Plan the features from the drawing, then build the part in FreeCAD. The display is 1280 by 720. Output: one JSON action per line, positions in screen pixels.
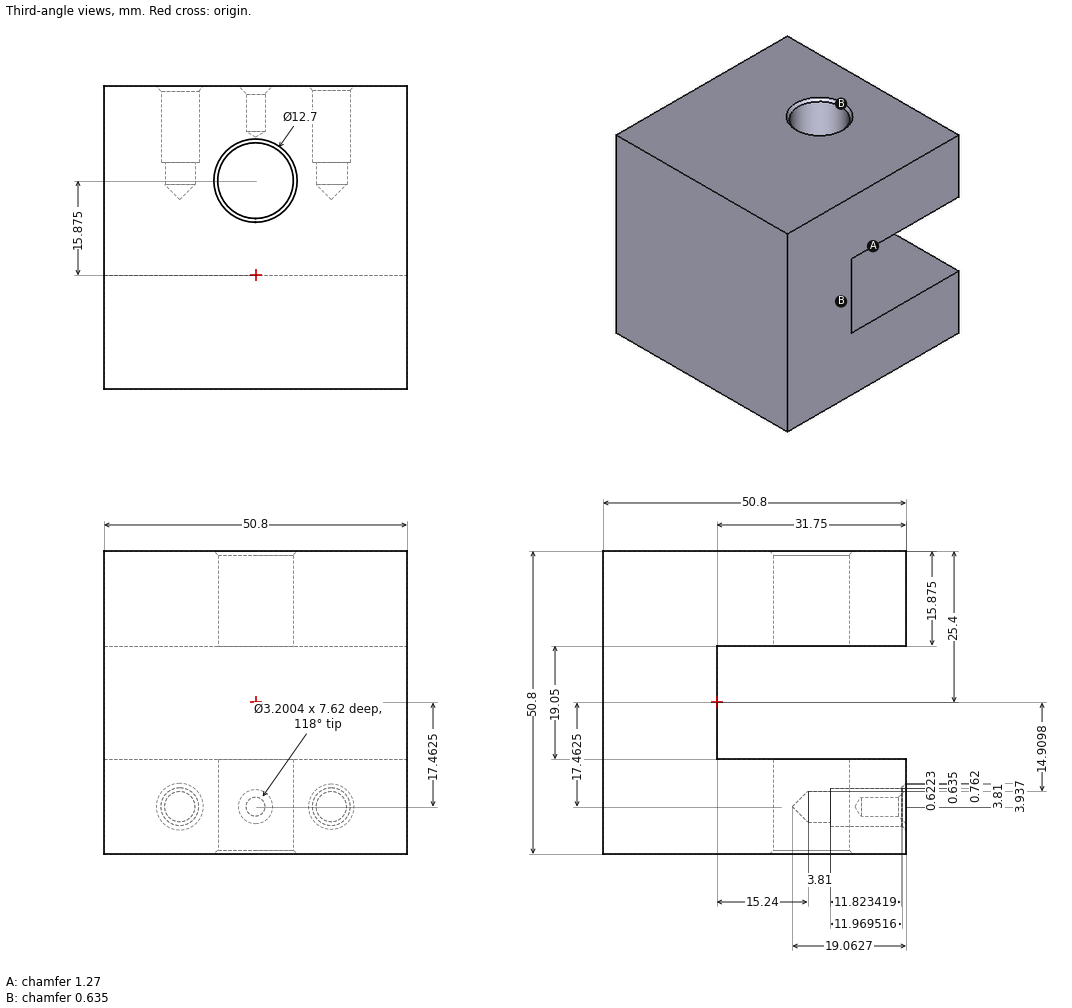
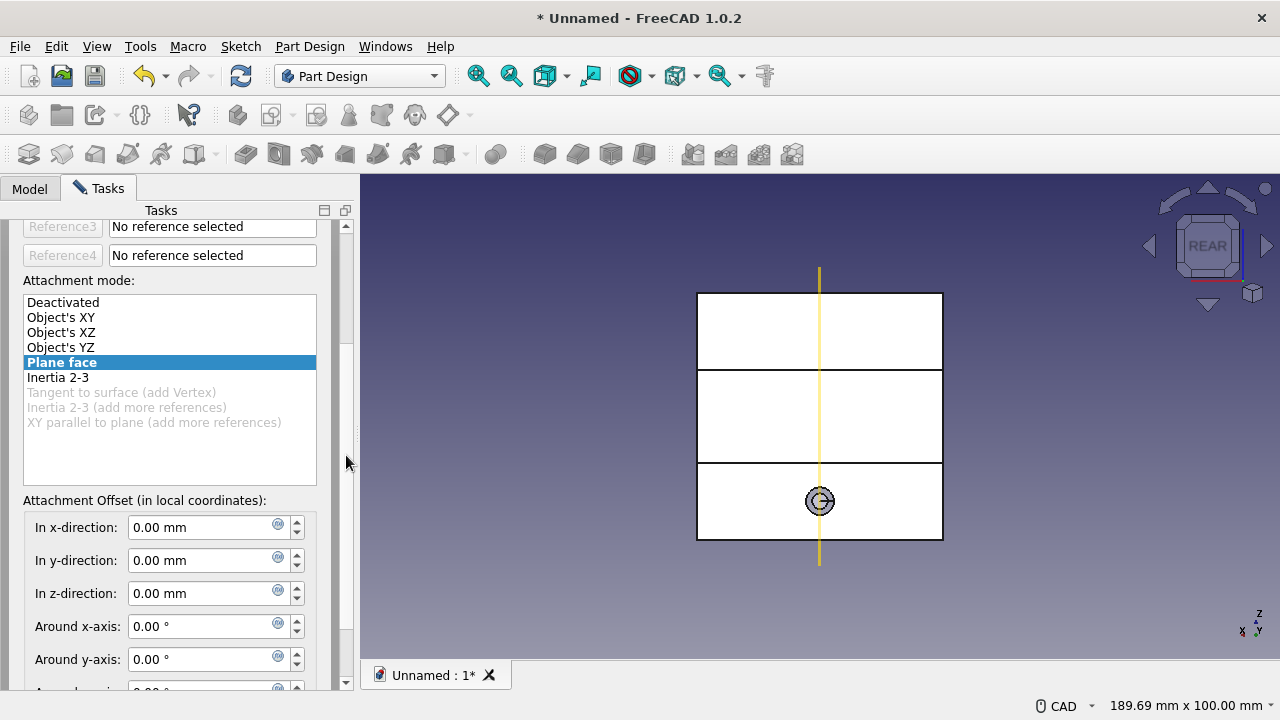
{"action": "triple_click", "coordinate": [210, 594]}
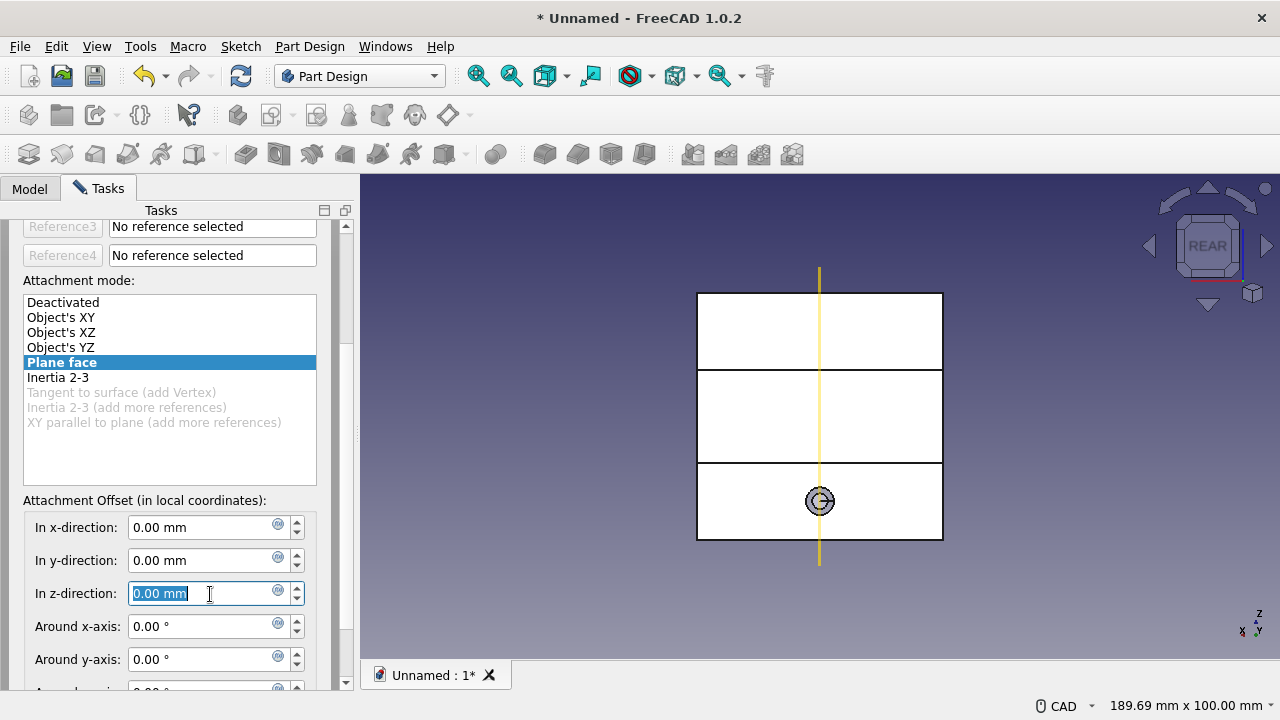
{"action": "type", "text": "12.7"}
{"action": "key", "text": "Tab"}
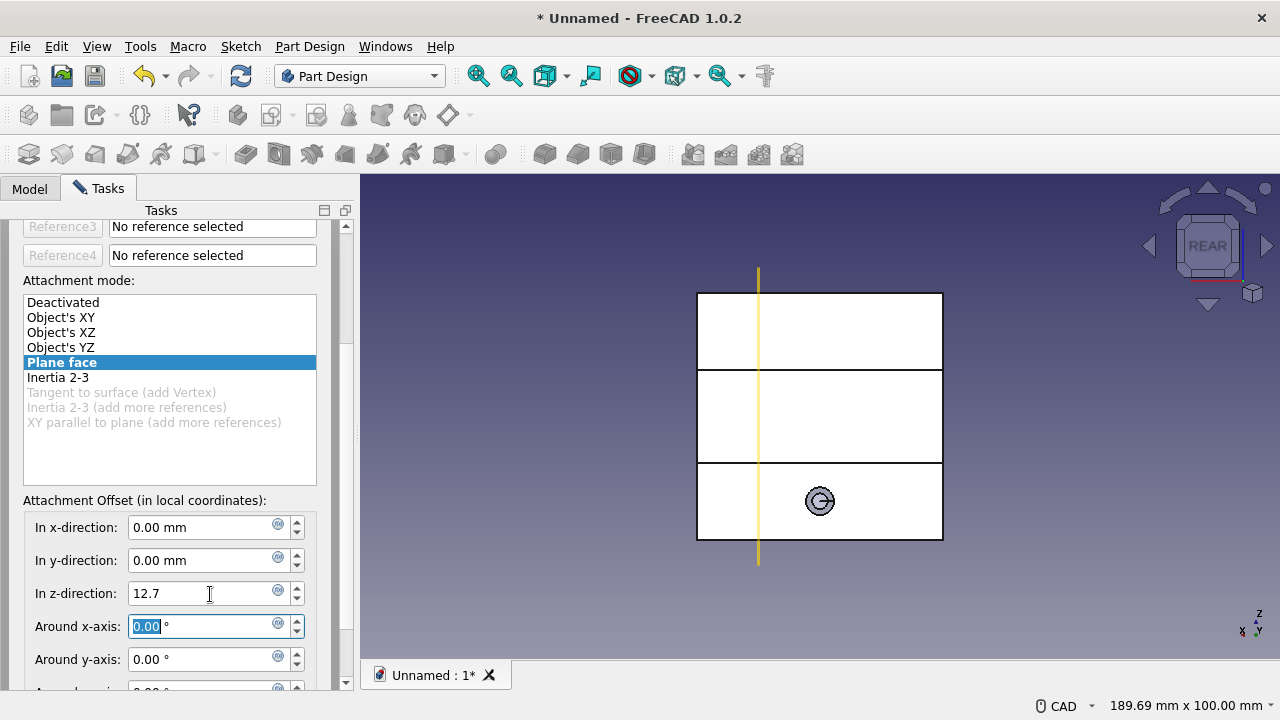
{"action": "scroll", "coordinate": [346, 455], "scroll_direction": "up", "scroll_amount": 4}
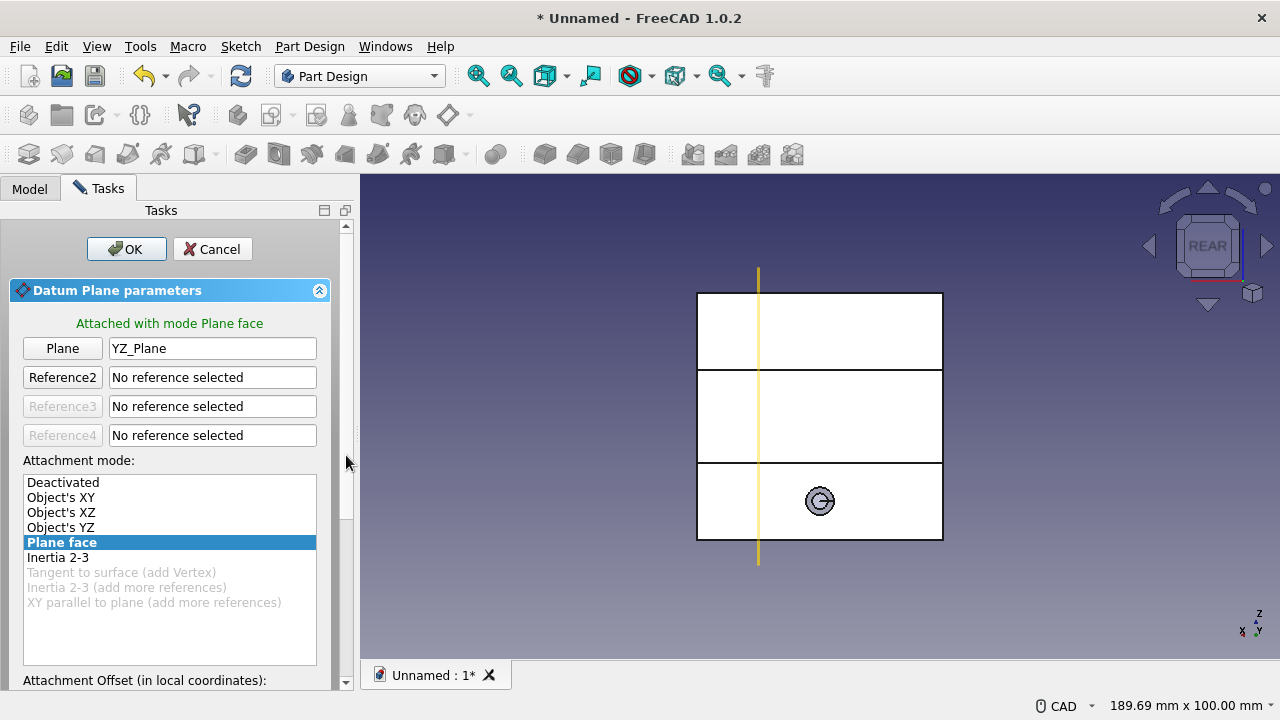
{"action": "left_click", "coordinate": [127, 249]}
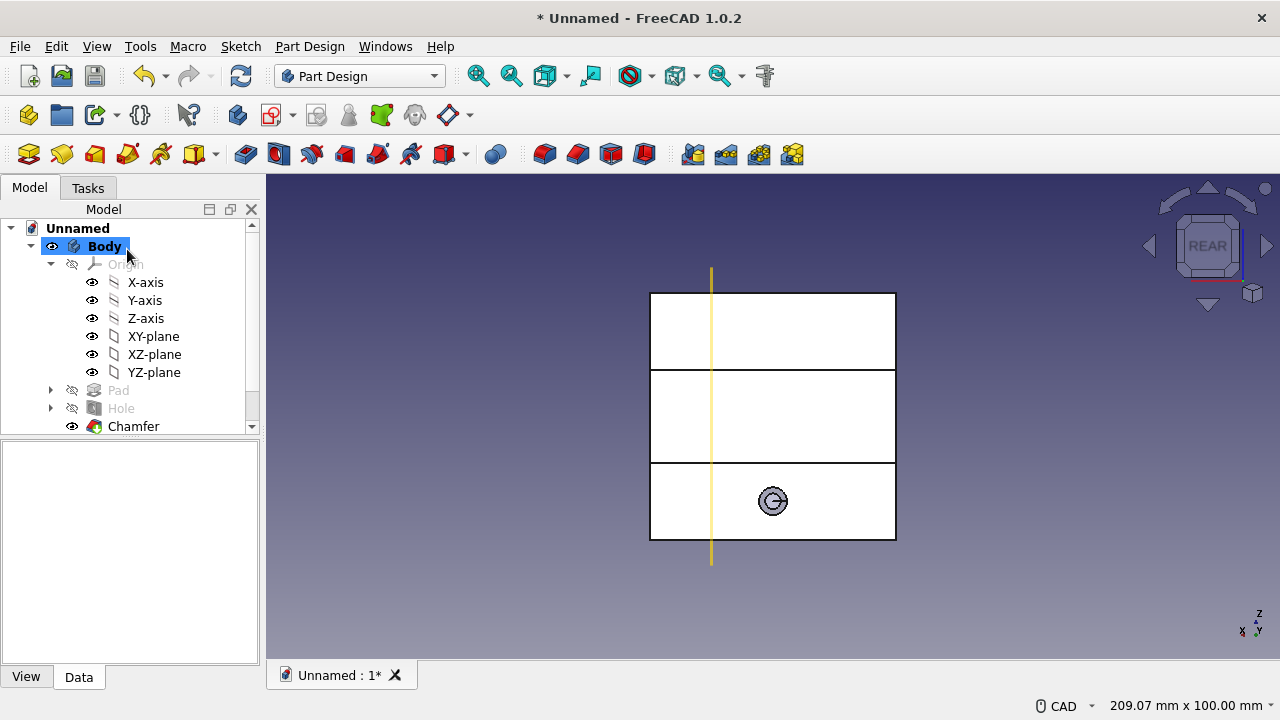
{"action": "scroll", "coordinate": [101, 332], "scroll_direction": "down", "scroll_amount": 3}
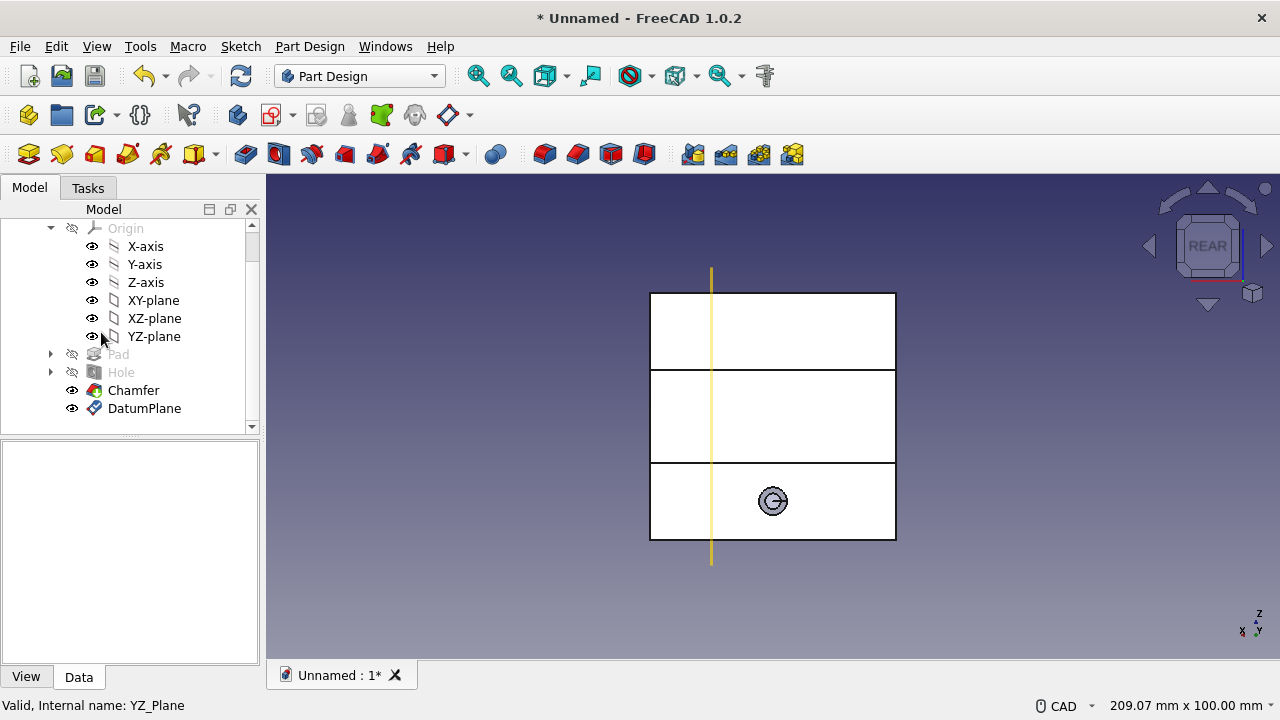
{"action": "left_click", "coordinate": [117, 408]}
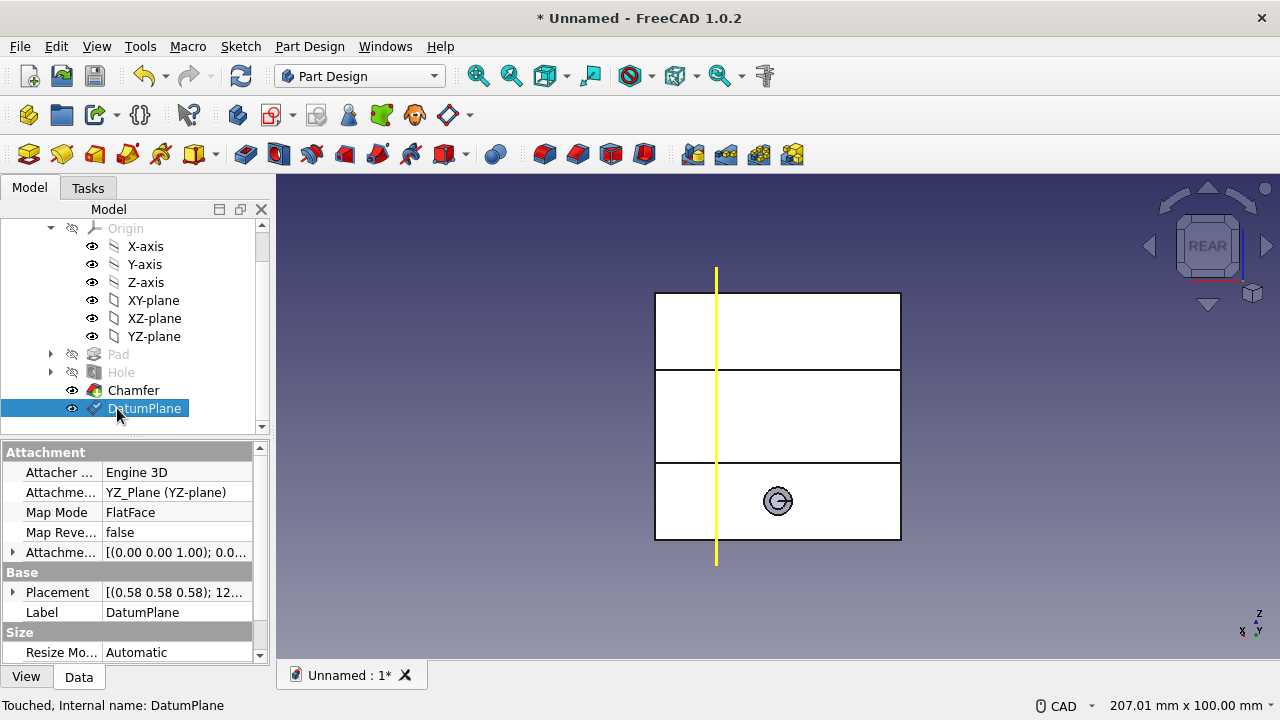
{"action": "left_click", "coordinate": [270, 116]}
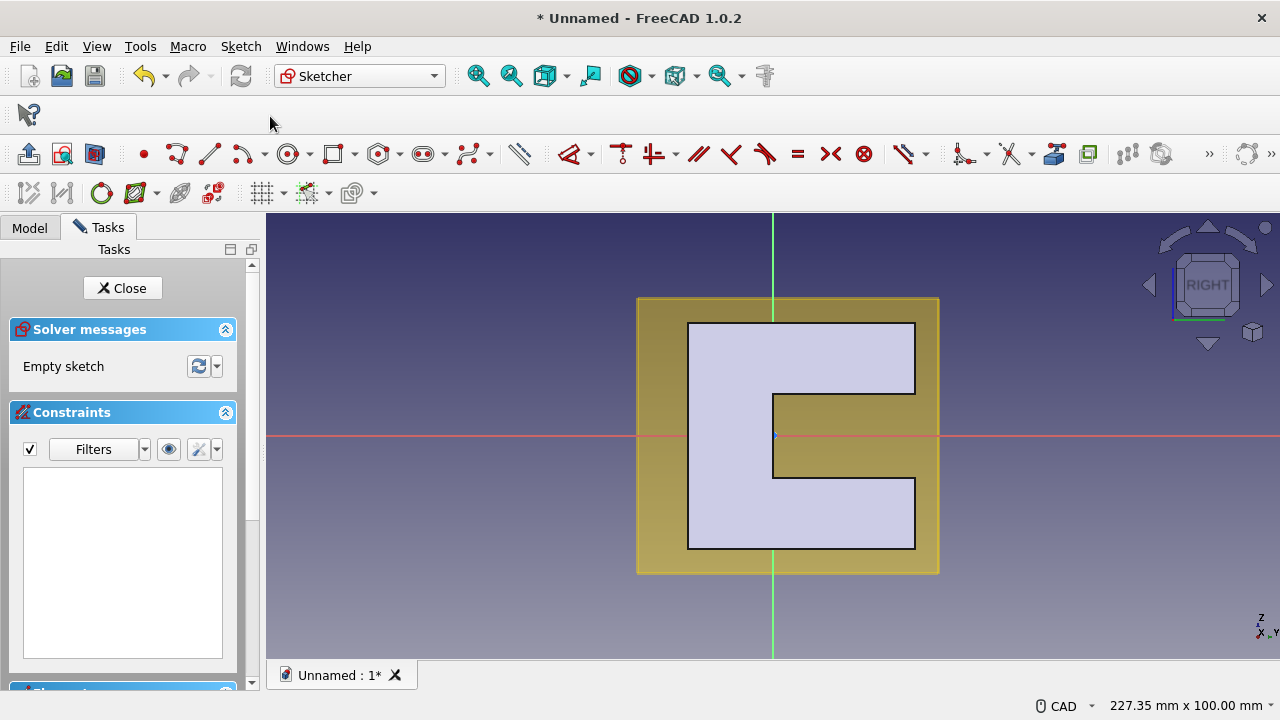
{"action": "left_click", "coordinate": [95, 154]}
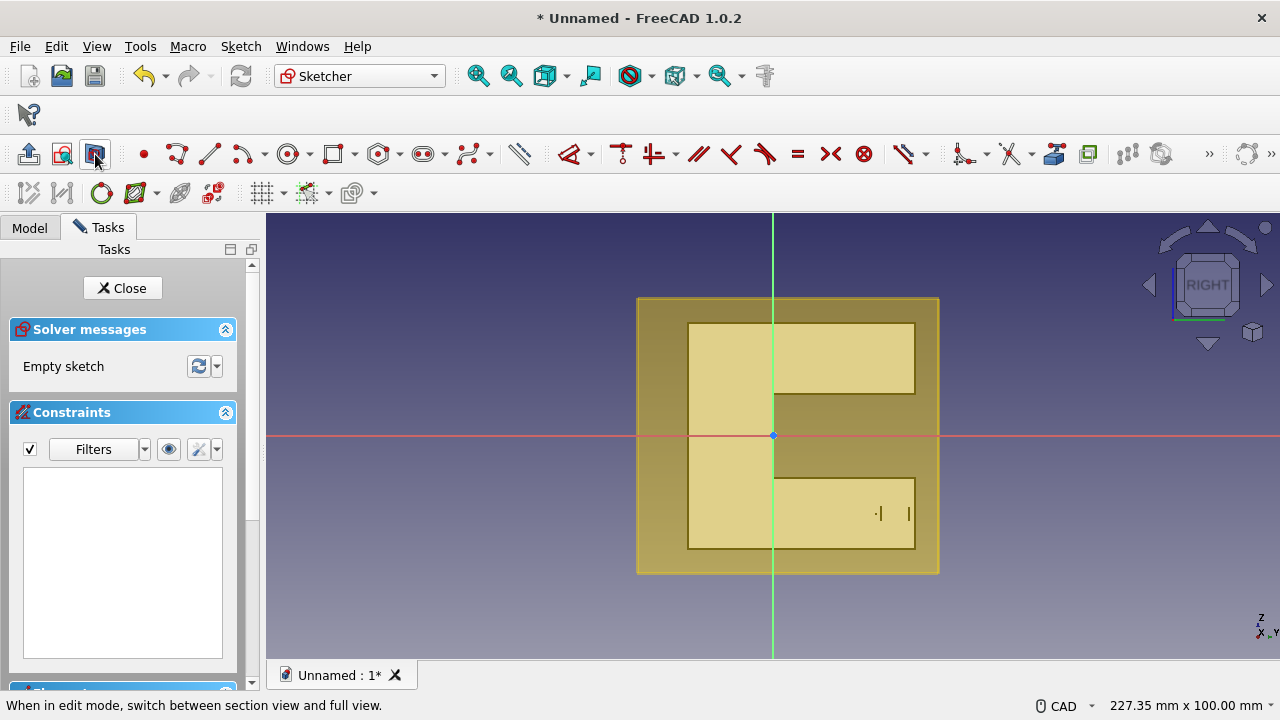
{"action": "scroll", "coordinate": [904, 492], "scroll_direction": "up", "scroll_amount": 6}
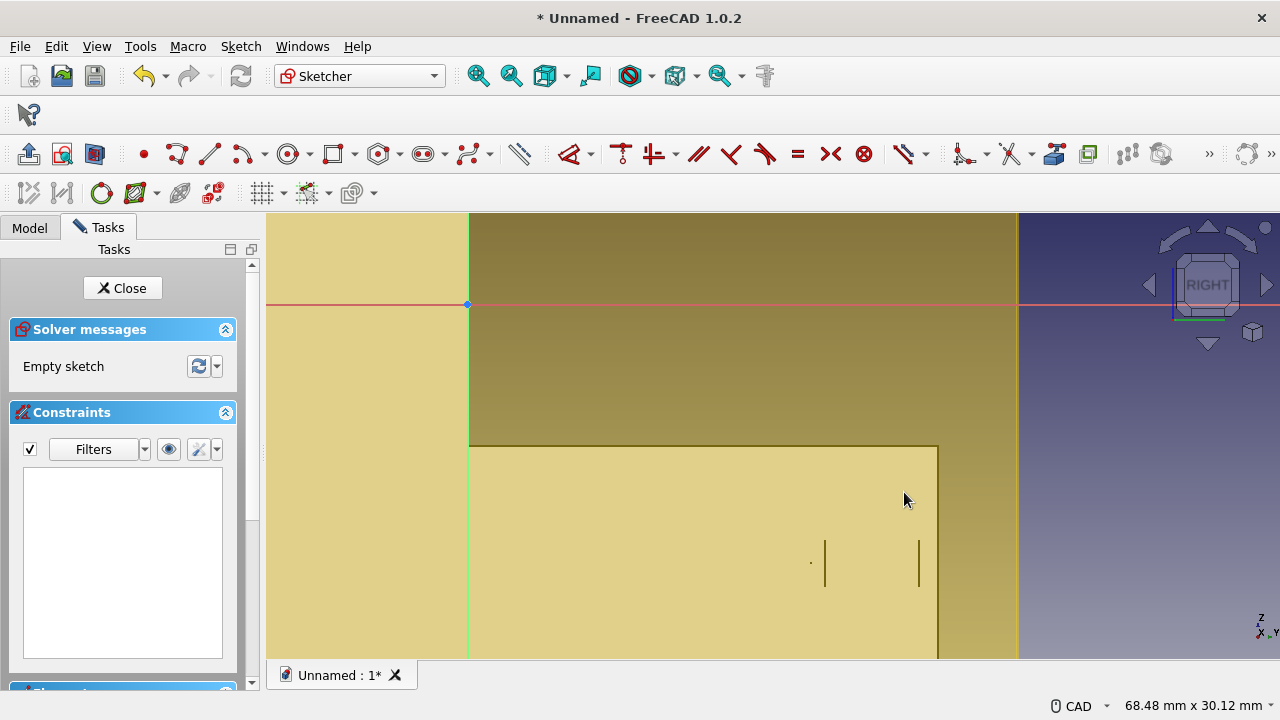
{"action": "left_click", "coordinate": [177, 154]}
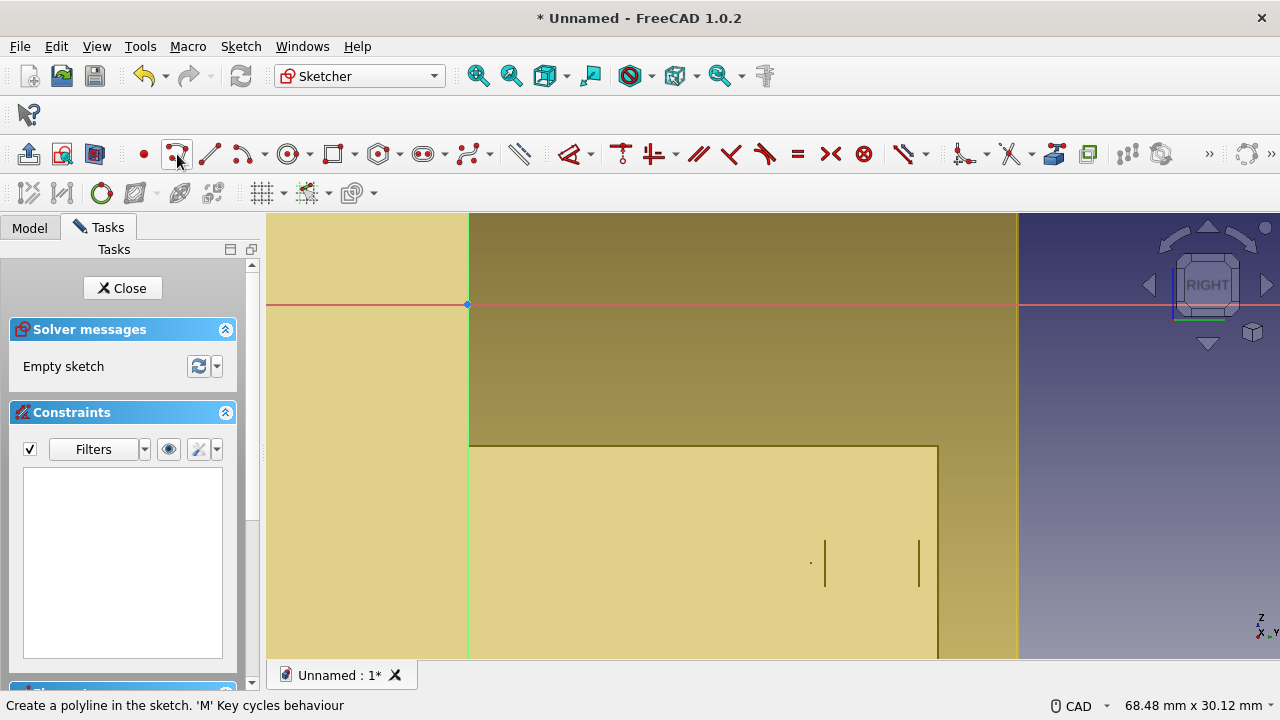
{"action": "left_click", "coordinate": [693, 525]}
{"action": "left_click", "coordinate": [655, 563]}
{"action": "left_click", "coordinate": [938, 563]}
{"action": "left_click", "coordinate": [938, 507]}